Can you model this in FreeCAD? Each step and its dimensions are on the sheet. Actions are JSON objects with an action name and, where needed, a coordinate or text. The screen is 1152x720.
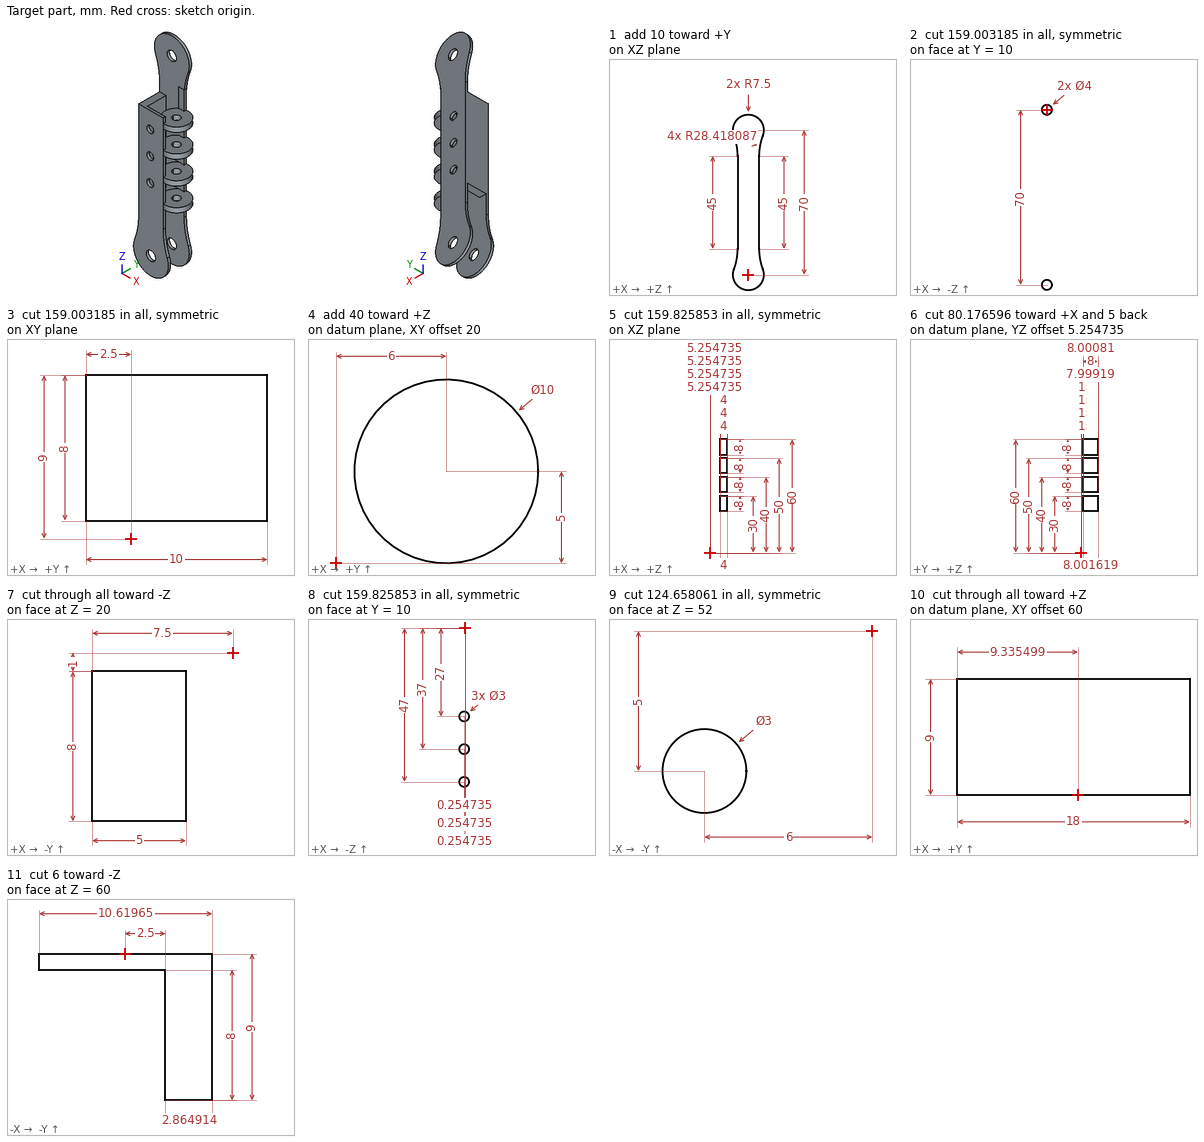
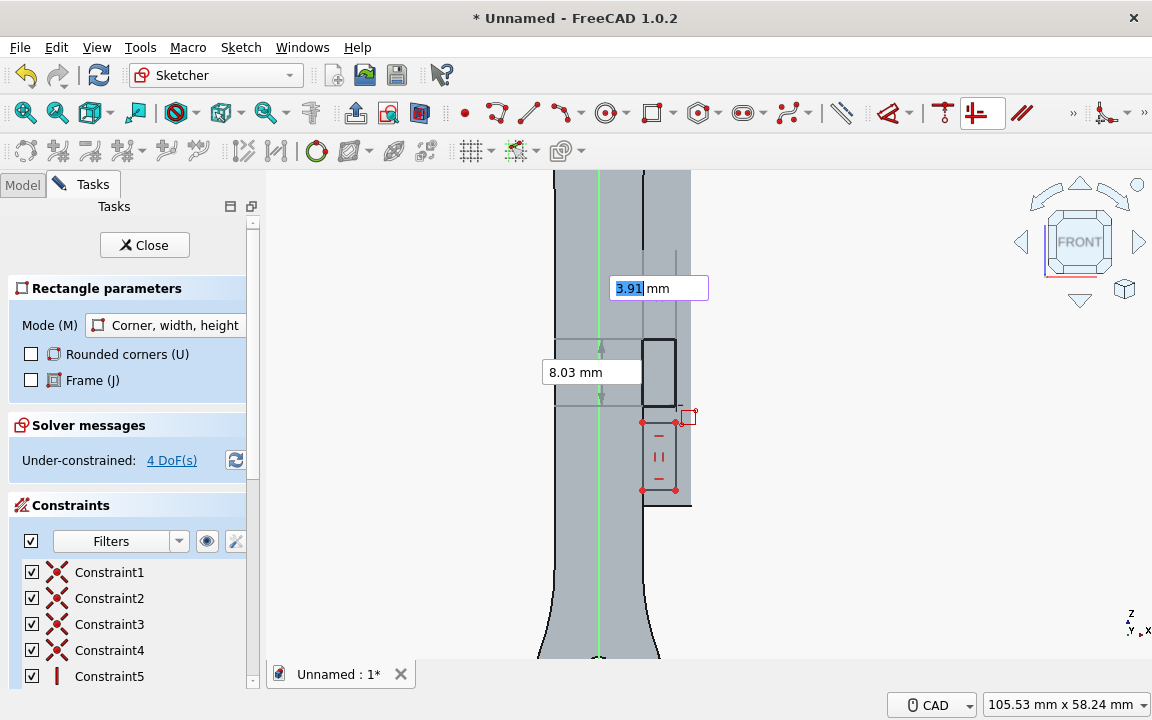
{"action": "left_click", "coordinate": [676, 405]}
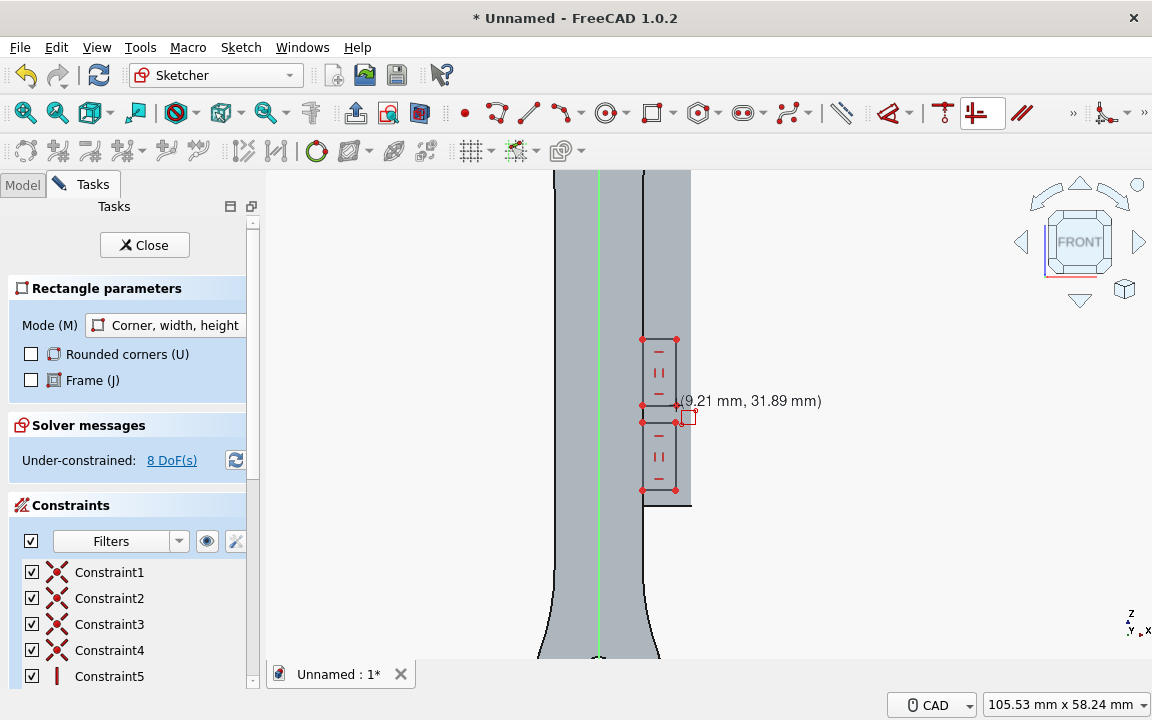
{"action": "left_click", "coordinate": [643, 254]}
{"action": "left_click", "coordinate": [676, 321]}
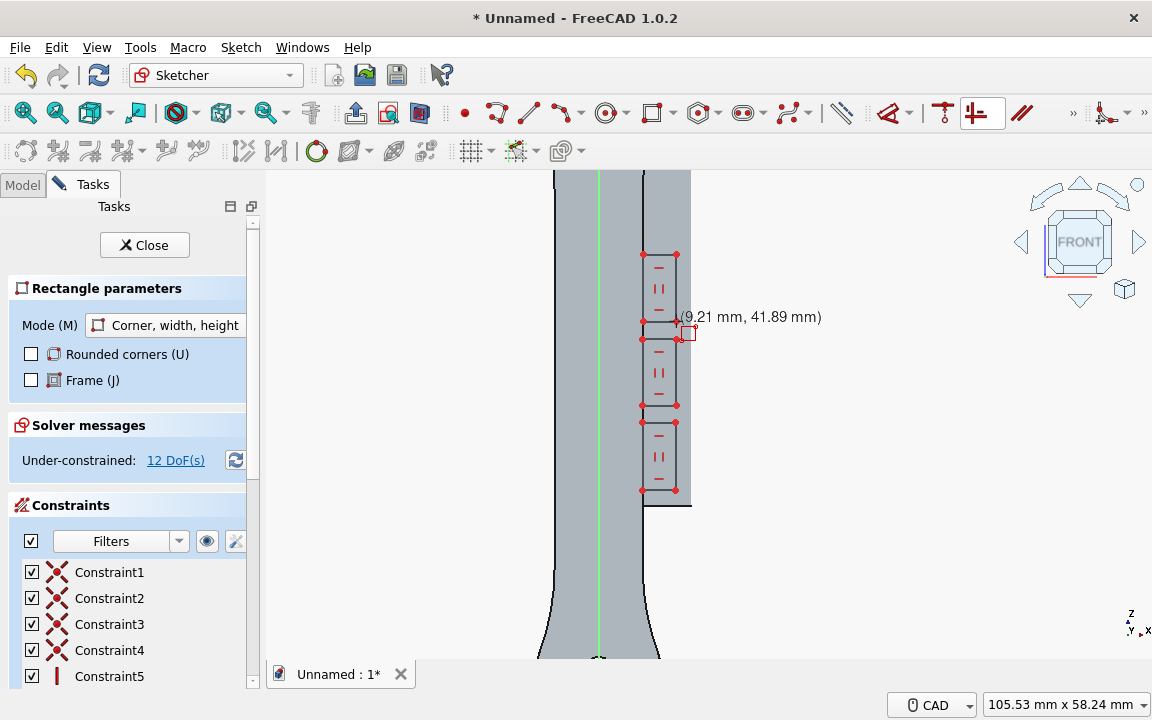
{"action": "scroll", "coordinate": [647, 400], "scroll_direction": "down", "scroll_amount": 2}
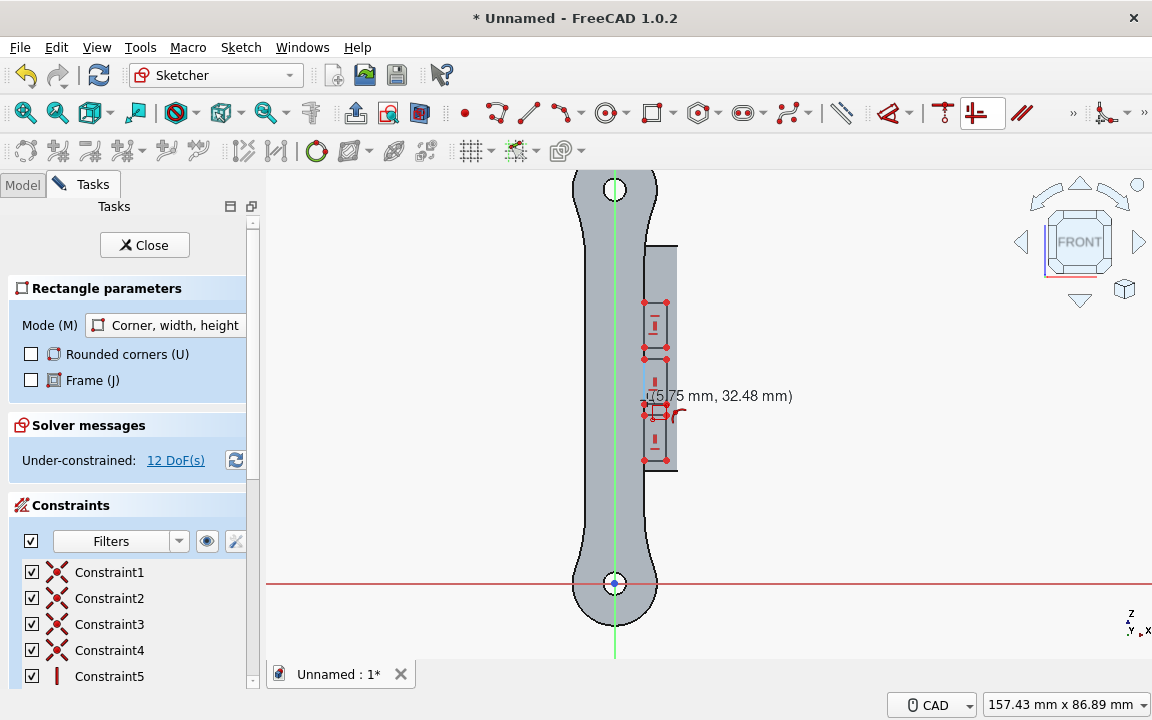
{"action": "left_click", "coordinate": [644, 246]}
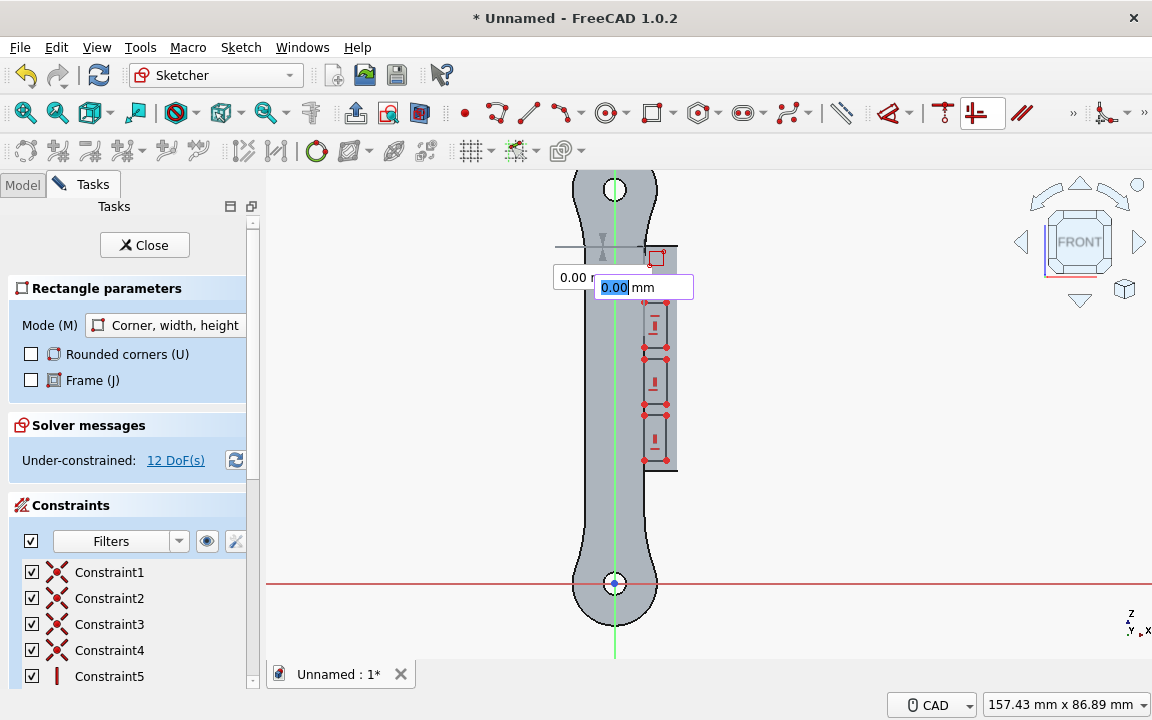
{"action": "scroll", "coordinate": [667, 291], "scroll_direction": "up", "scroll_amount": 2}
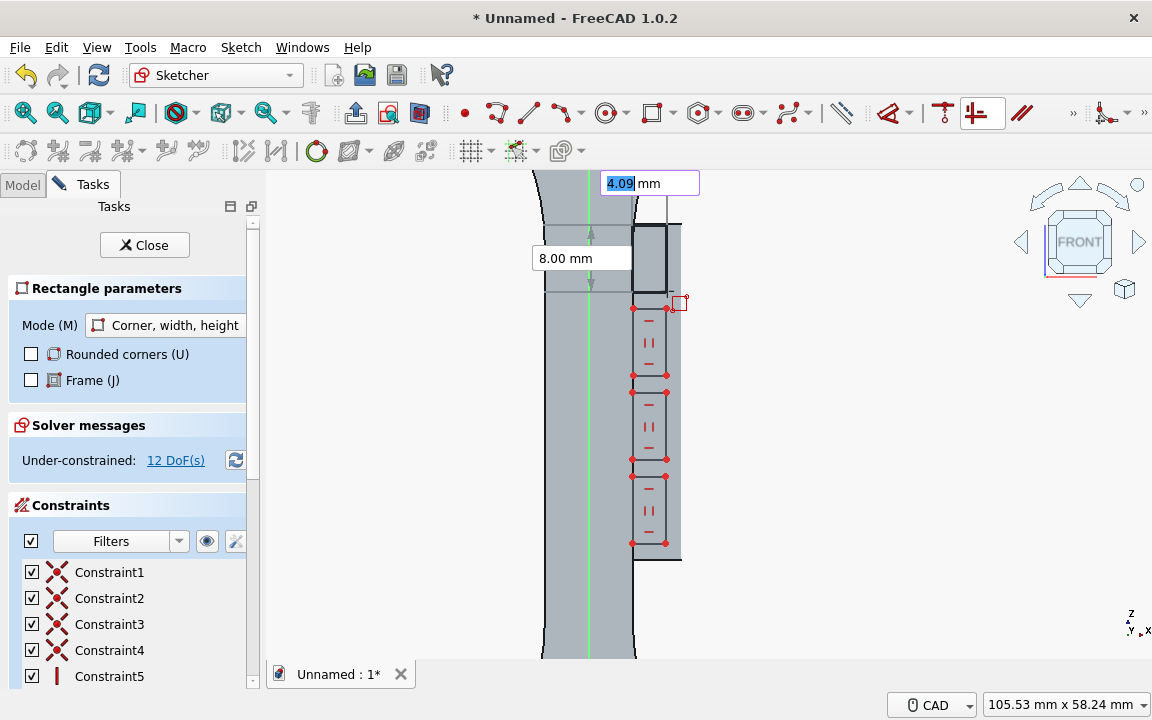
{"action": "left_click", "coordinate": [667, 291]}
{"action": "key", "text": "Escape"}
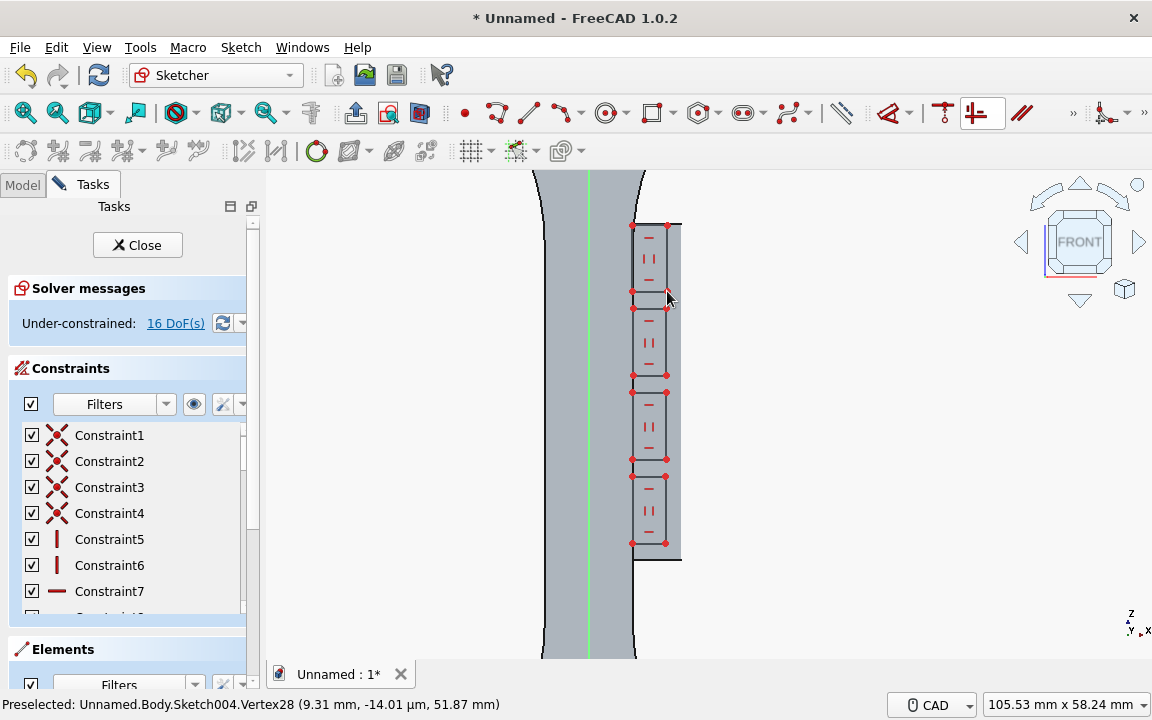
{"action": "key", "text": "d"}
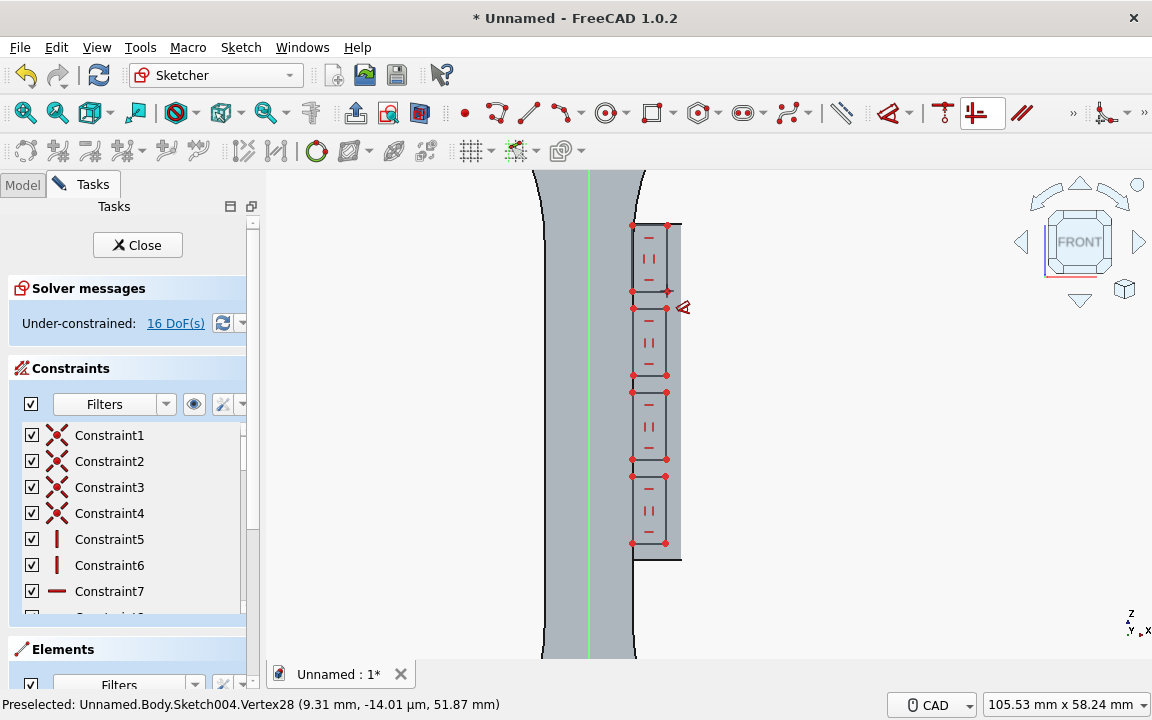
{"action": "left_click", "coordinate": [633, 497]}
{"action": "left_click", "coordinate": [691, 510]}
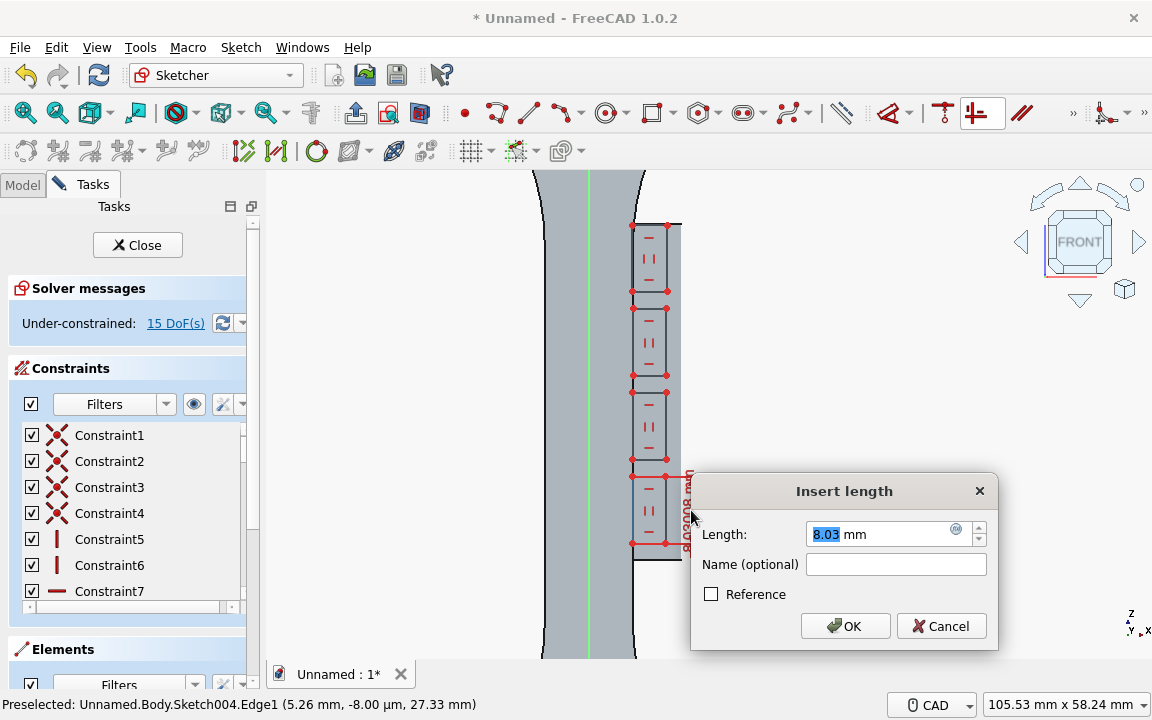
{"action": "type", "text": "8"}
{"action": "key", "text": "Return"}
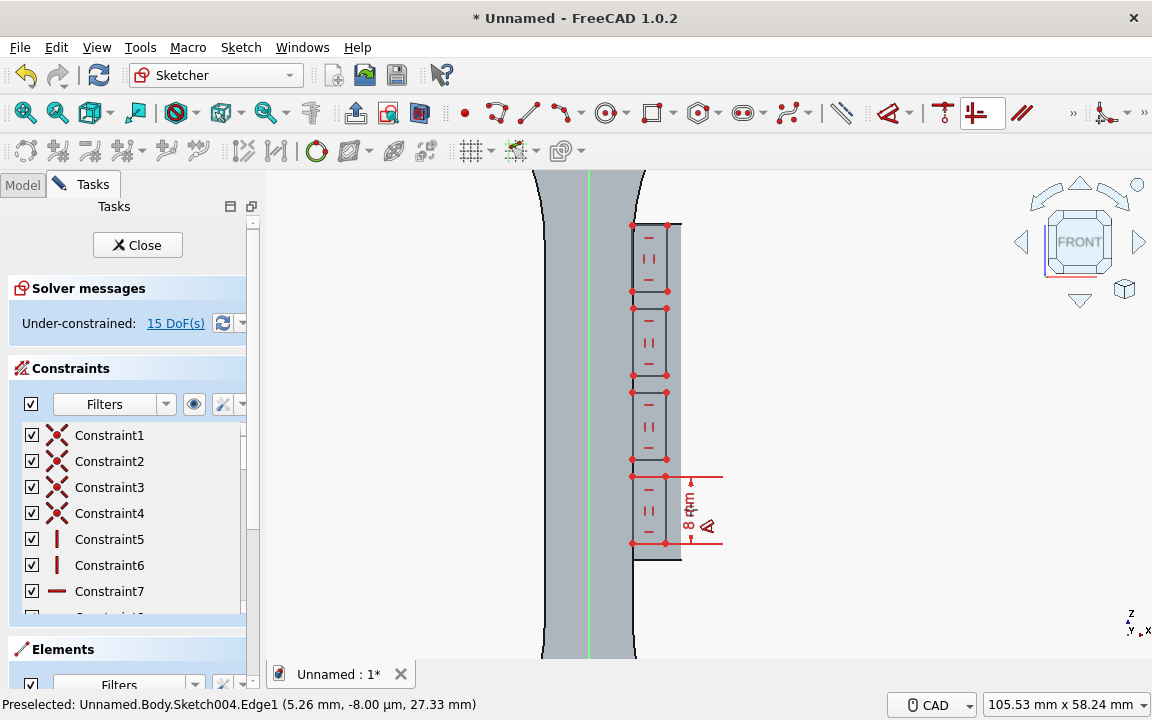
{"action": "scroll", "coordinate": [643, 544], "scroll_direction": "up", "scroll_amount": 2}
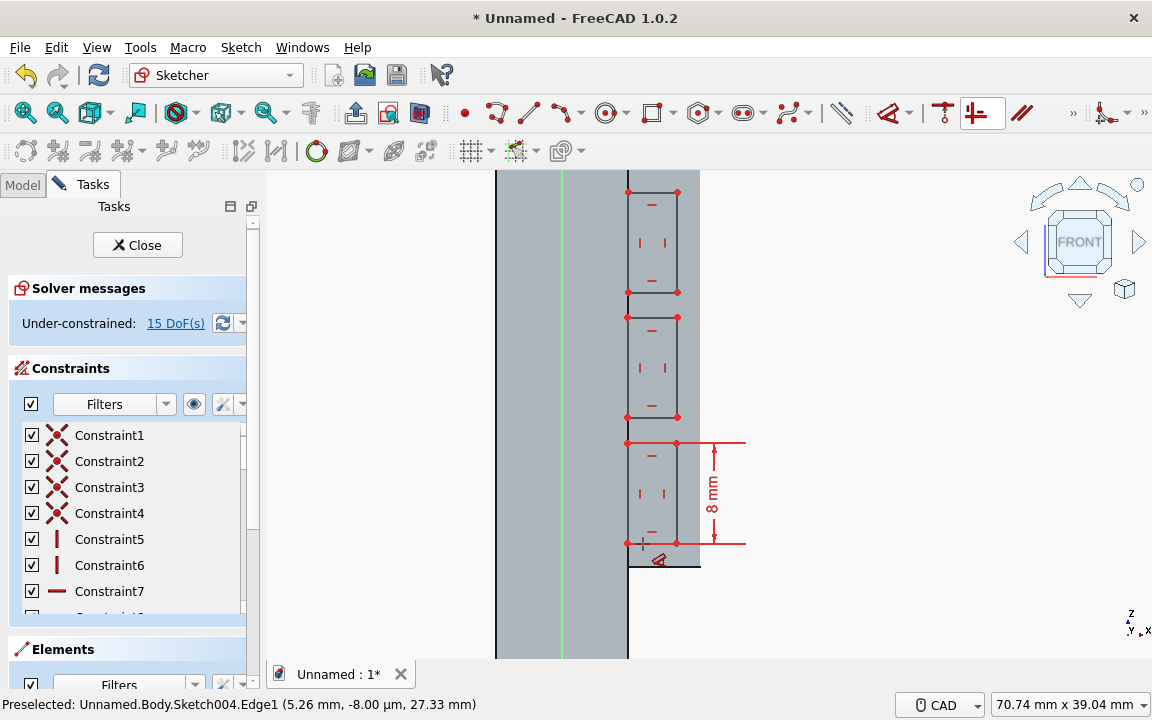
{"action": "left_click", "coordinate": [643, 544]}
{"action": "left_click", "coordinate": [652, 578]}